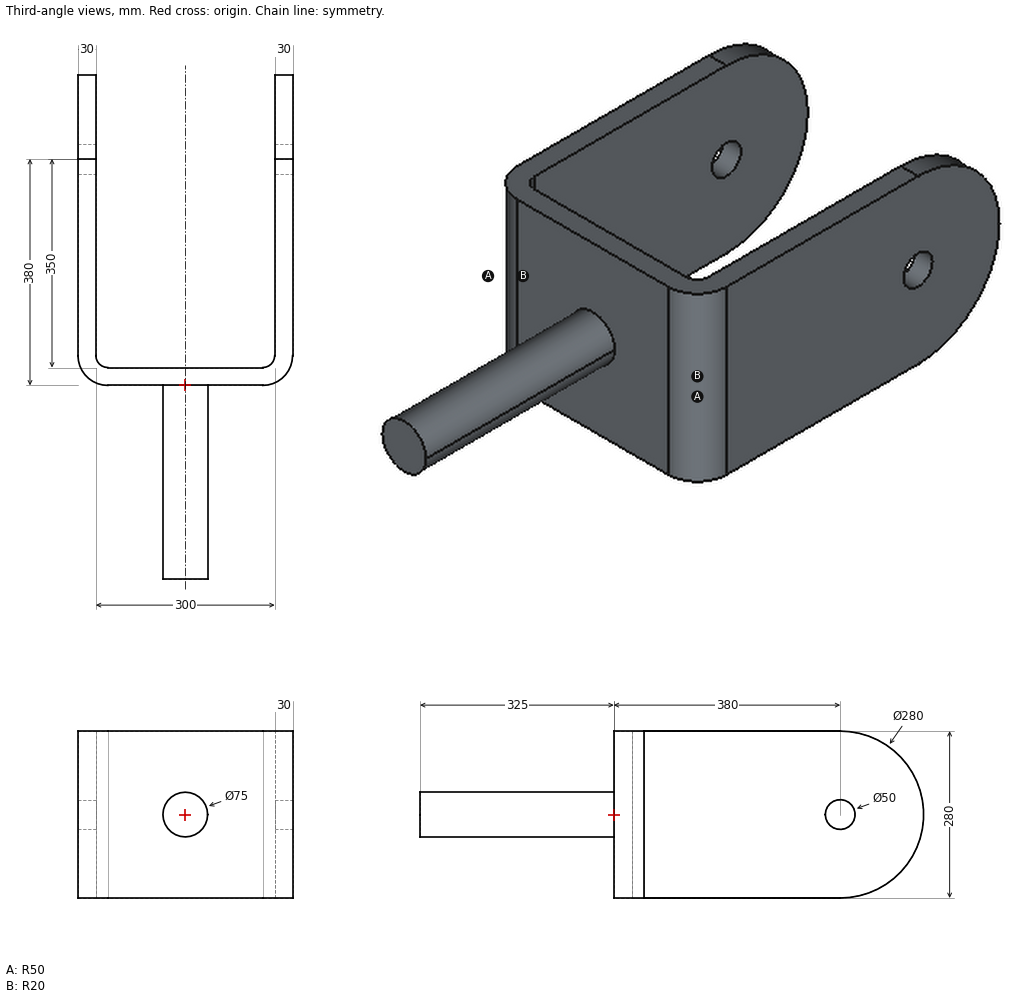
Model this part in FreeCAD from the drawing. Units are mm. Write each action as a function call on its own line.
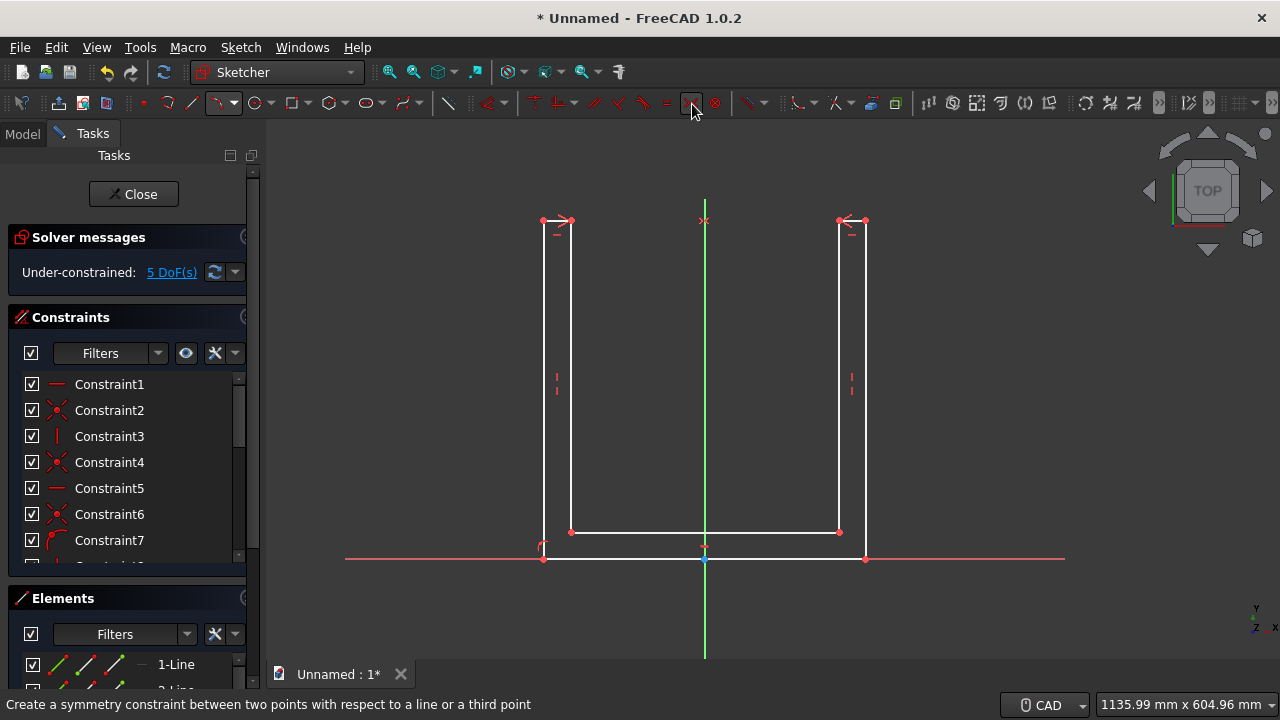
click(488, 104)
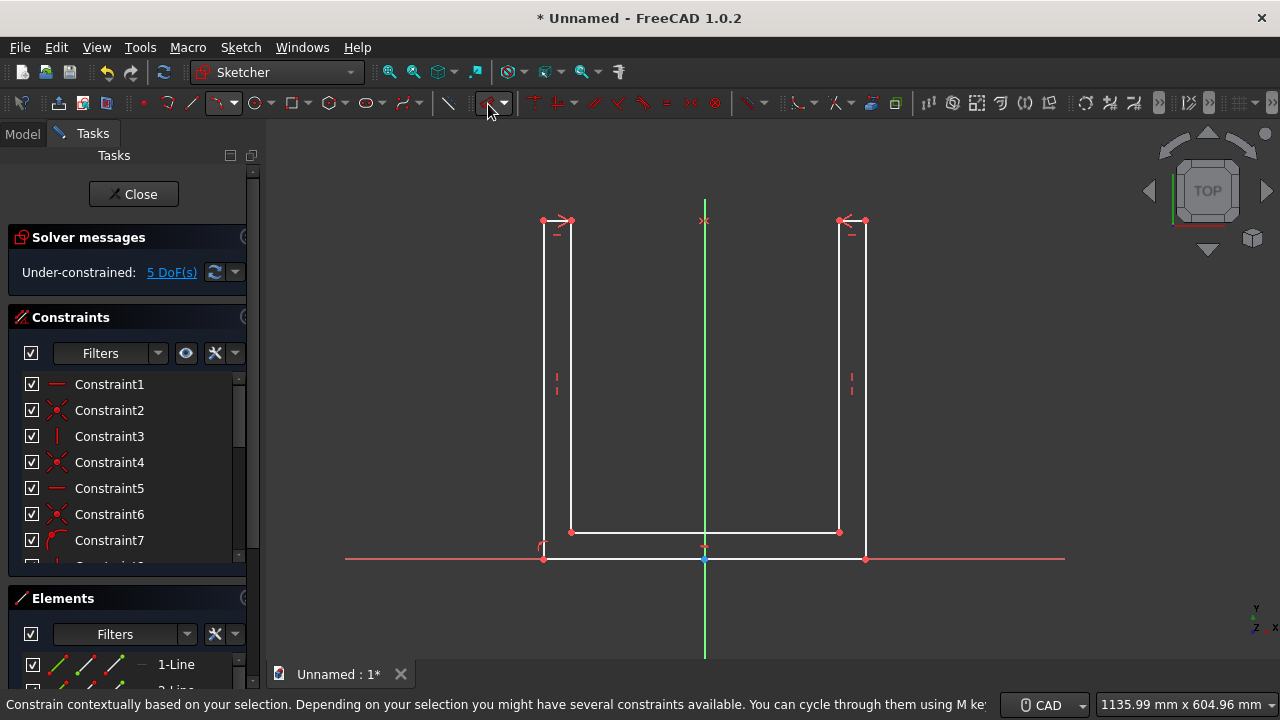
scroll(560, 221, up, 2)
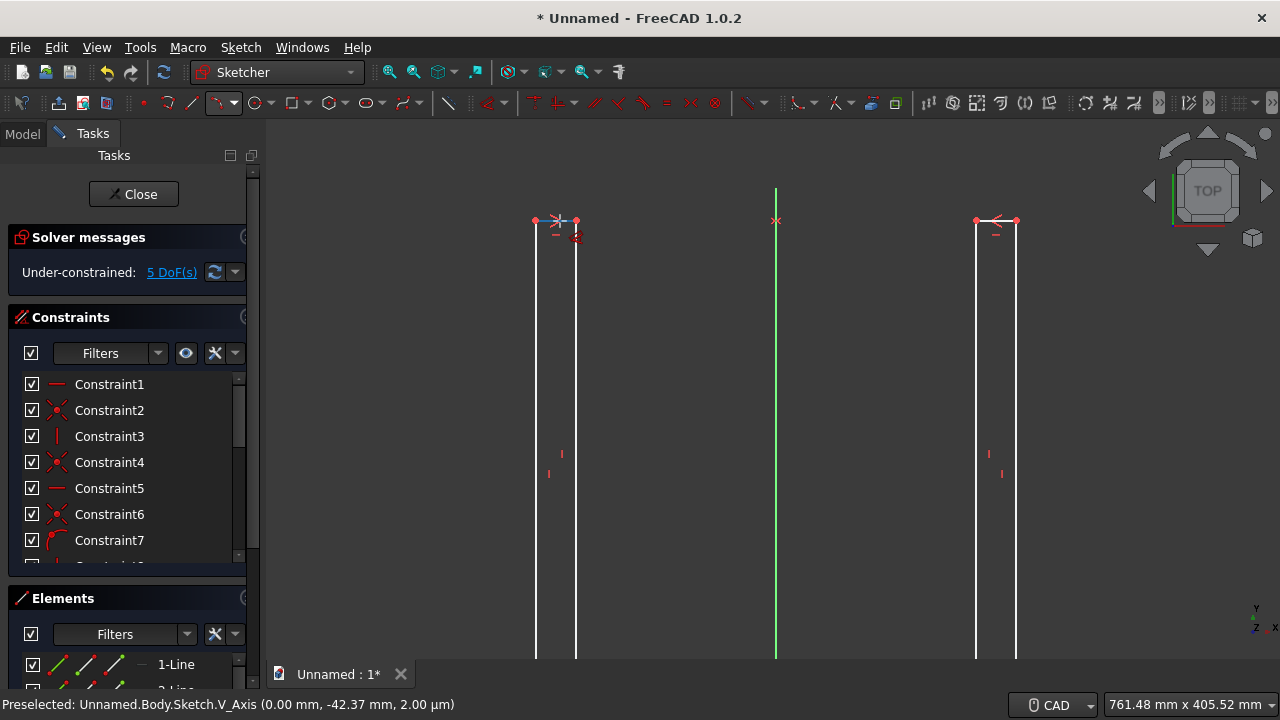
click(560, 221)
click(556, 187)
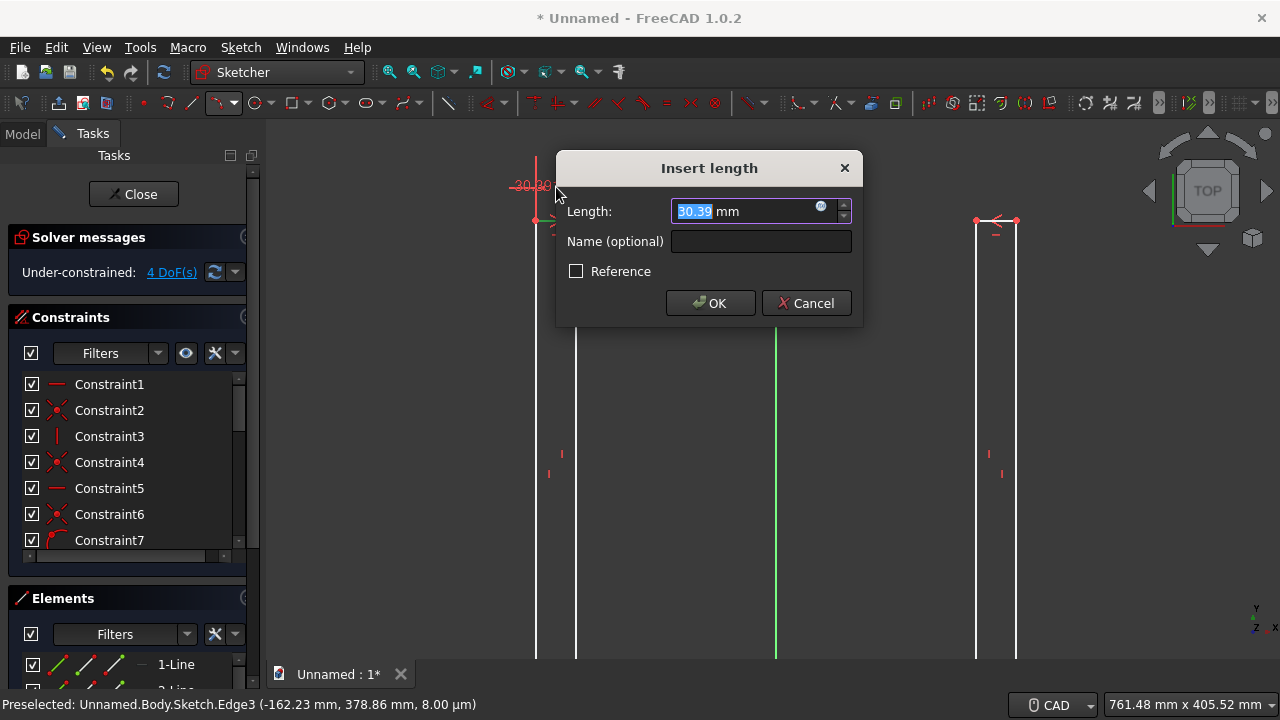
text(30)
key(Return)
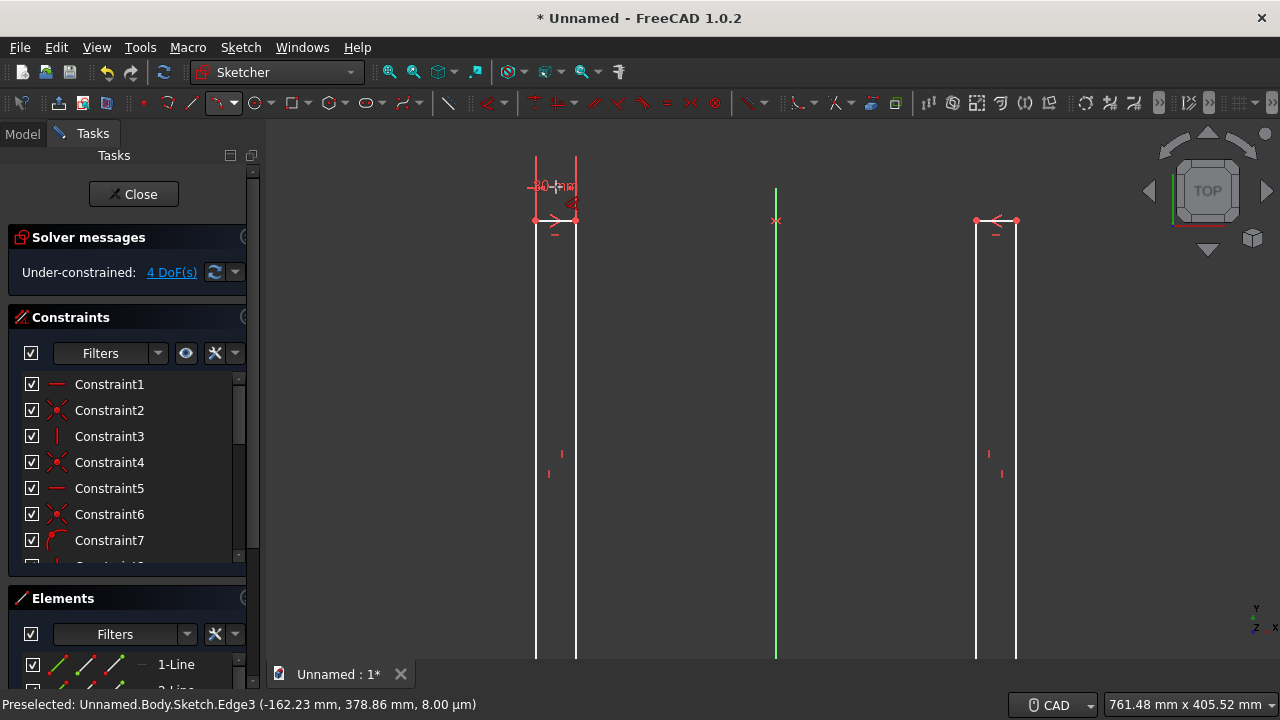
click(1004, 221)
click(996, 187)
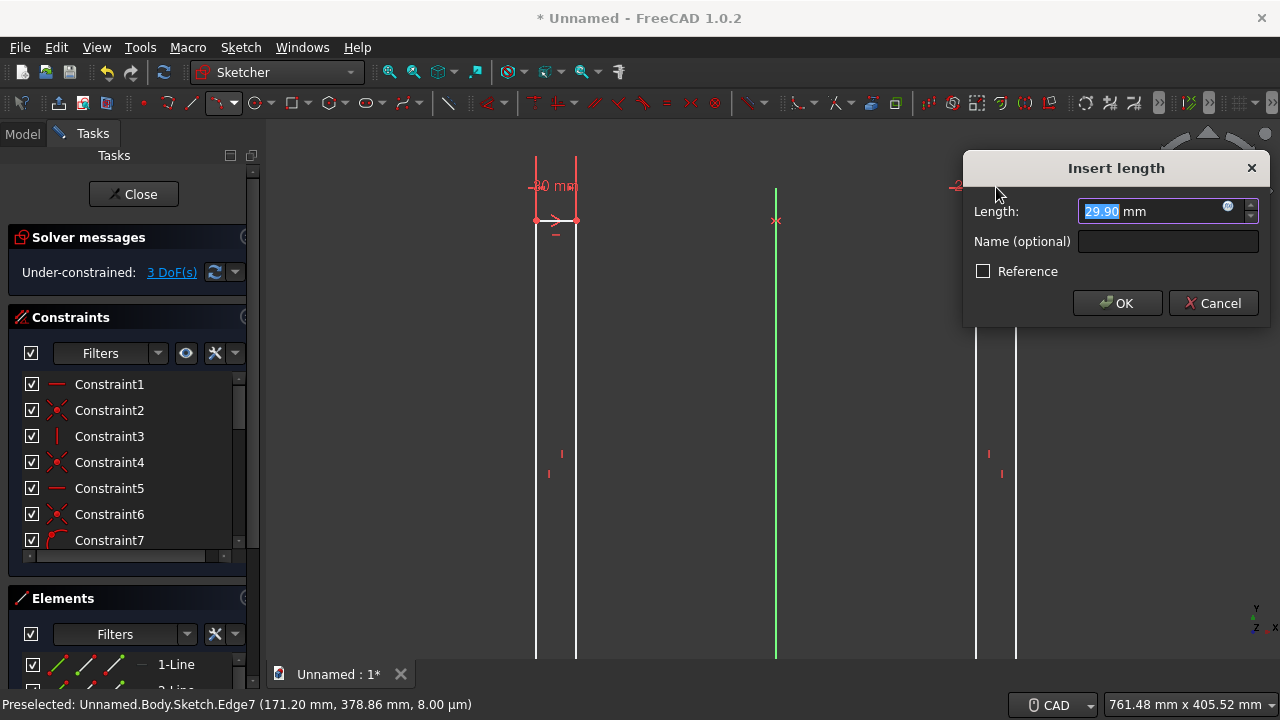
text(30)
key(Return)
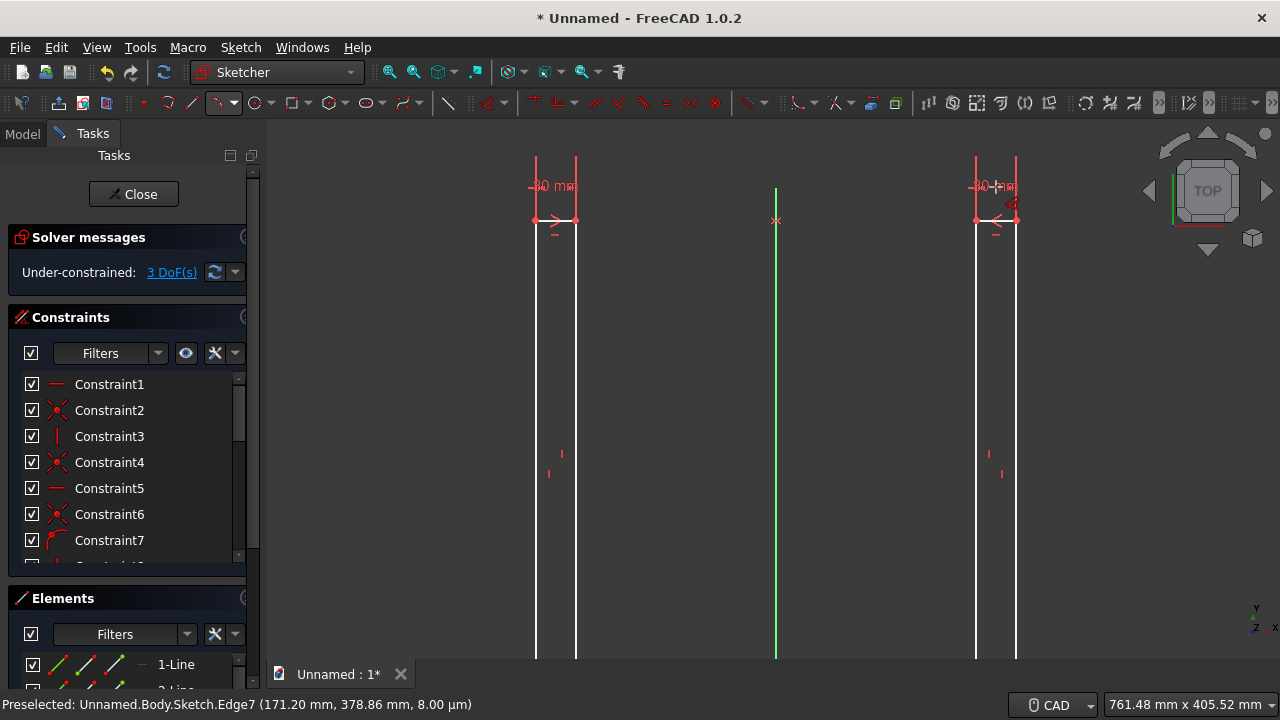
scroll(559, 219, down, 2)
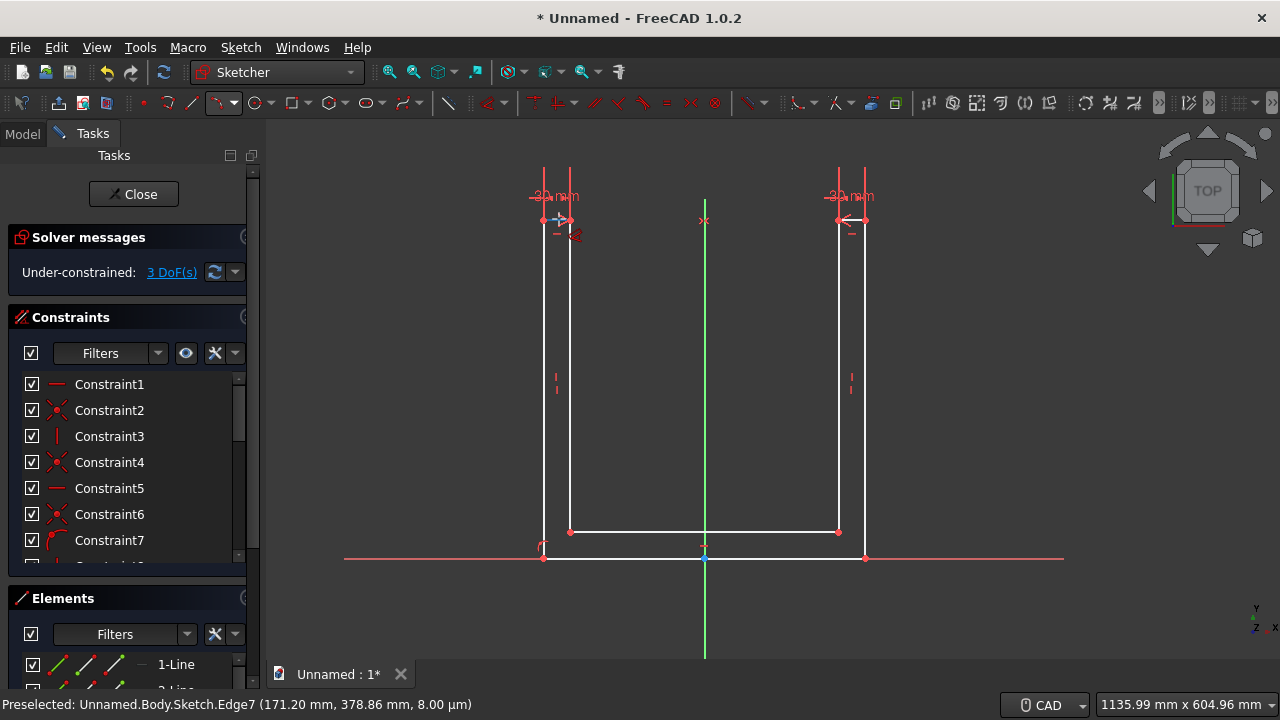
click(758, 532)
click(643, 498)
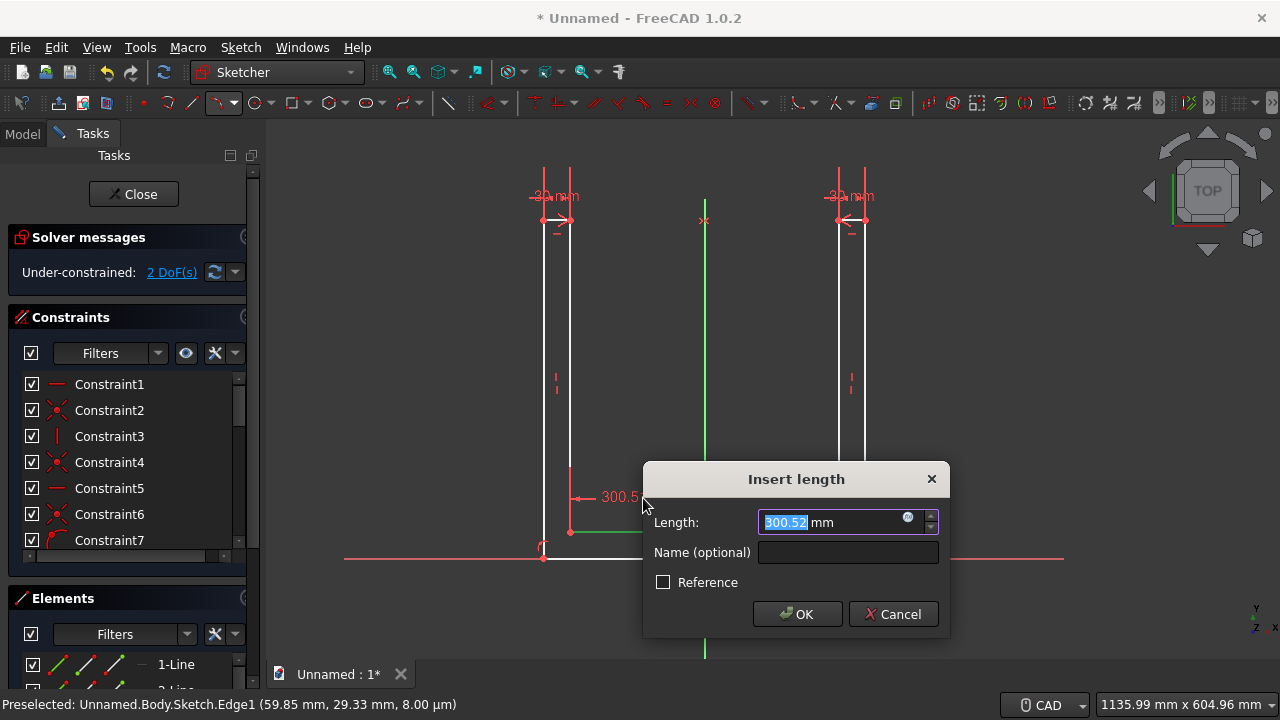
text(300)
key(Return)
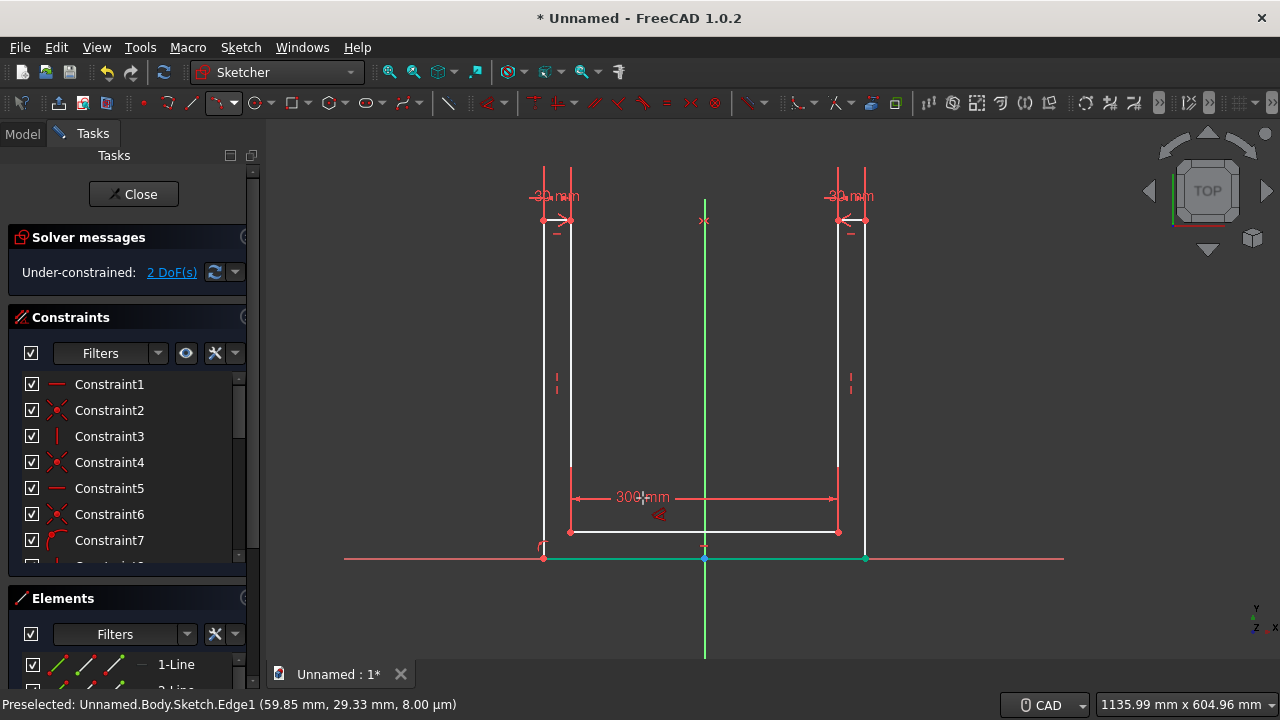
click(571, 439)
click(605, 376)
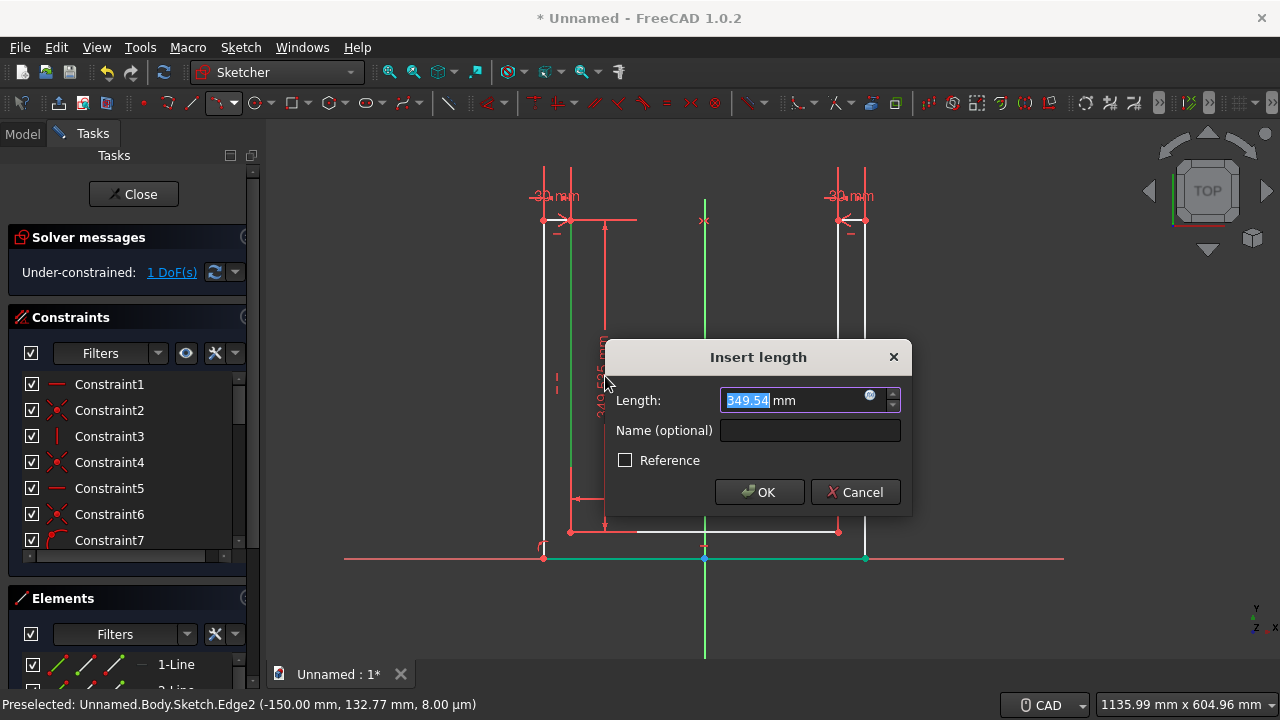
text(350)
key(Return)